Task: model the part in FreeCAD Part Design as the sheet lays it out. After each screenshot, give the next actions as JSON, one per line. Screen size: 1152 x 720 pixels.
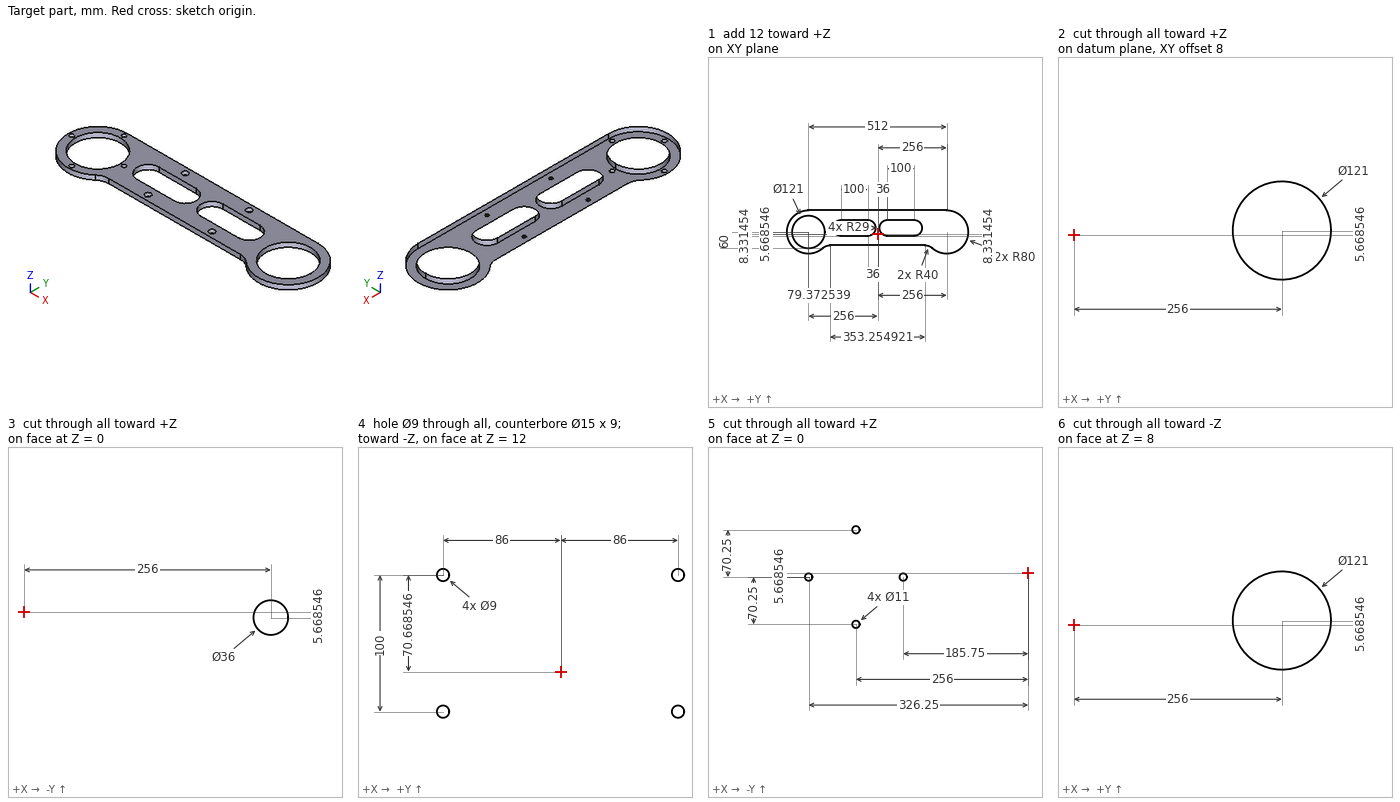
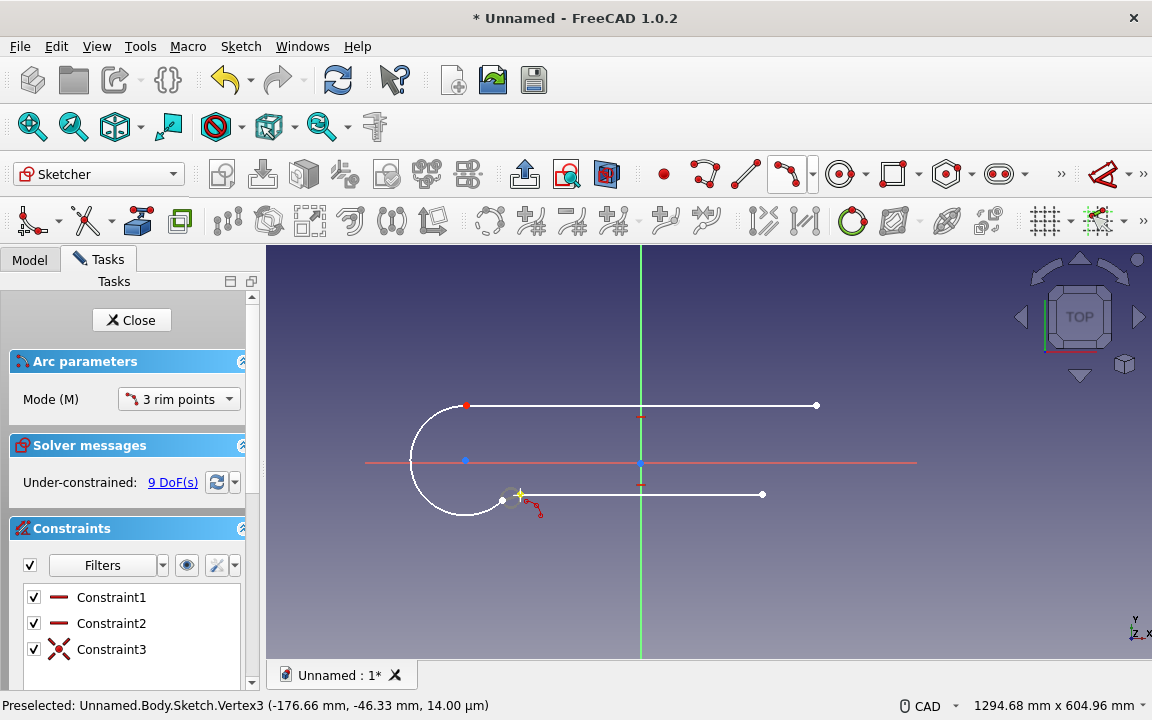
{"action": "scroll", "coordinate": [510, 495], "scroll_direction": "up", "scroll_amount": 11}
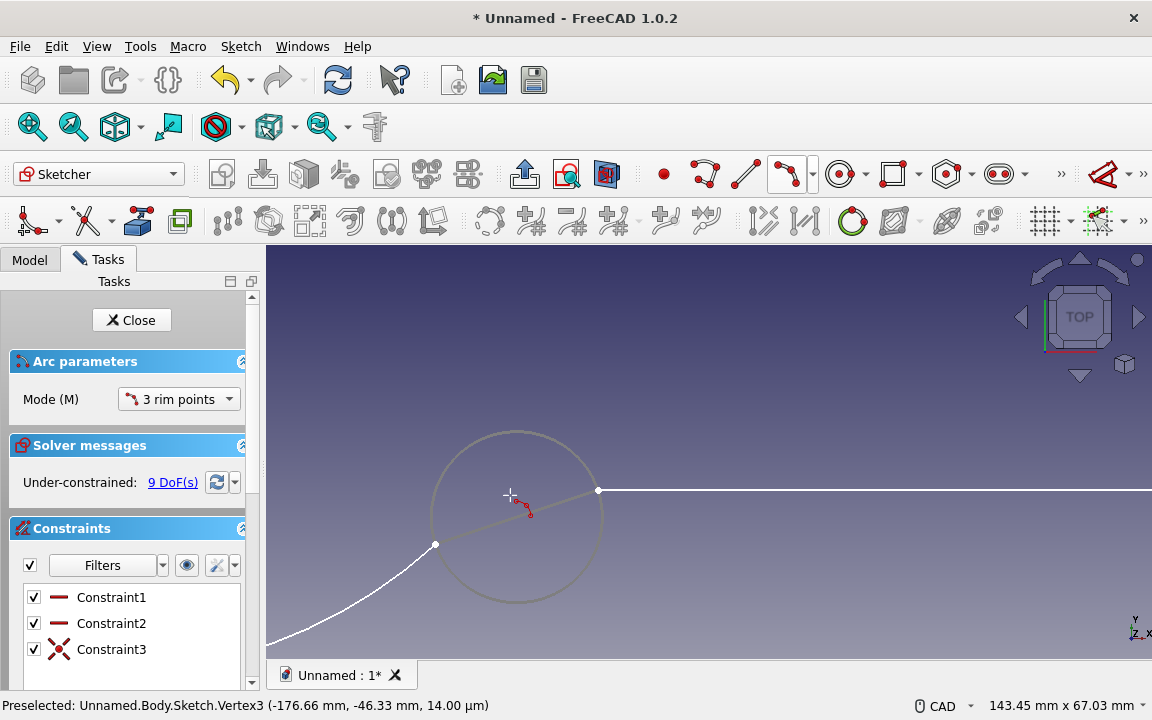
{"action": "left_click", "coordinate": [511, 494]}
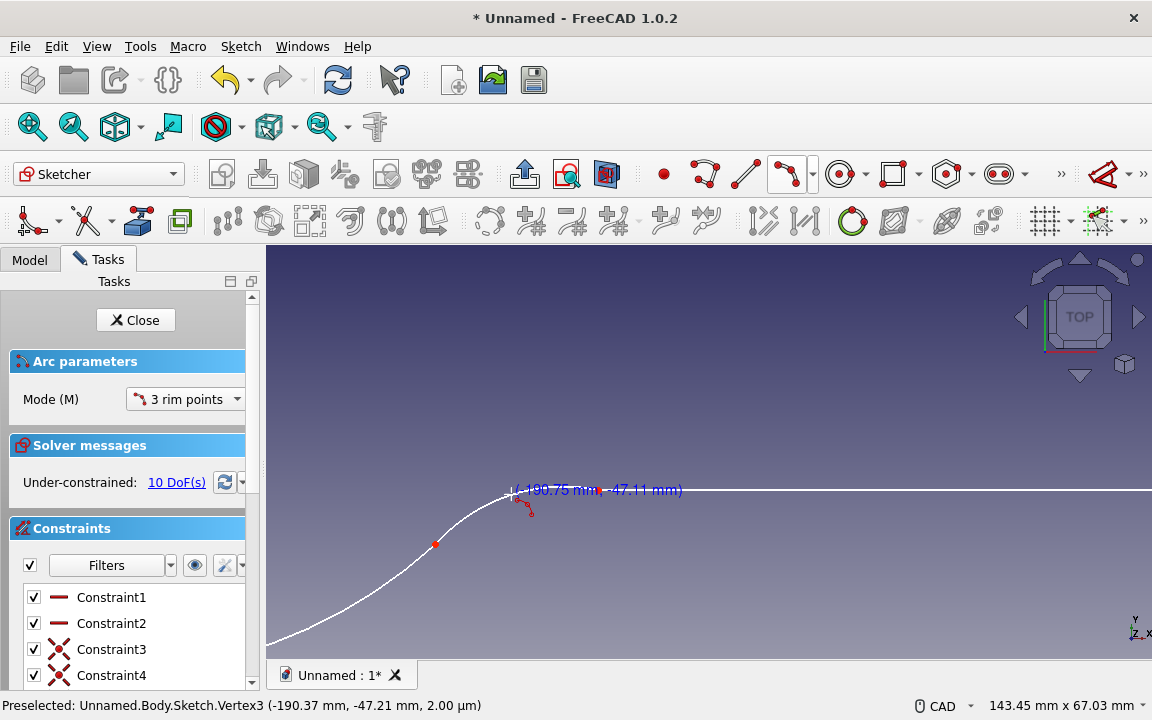
{"action": "scroll", "coordinate": [510, 495], "scroll_direction": "down", "scroll_amount": 11}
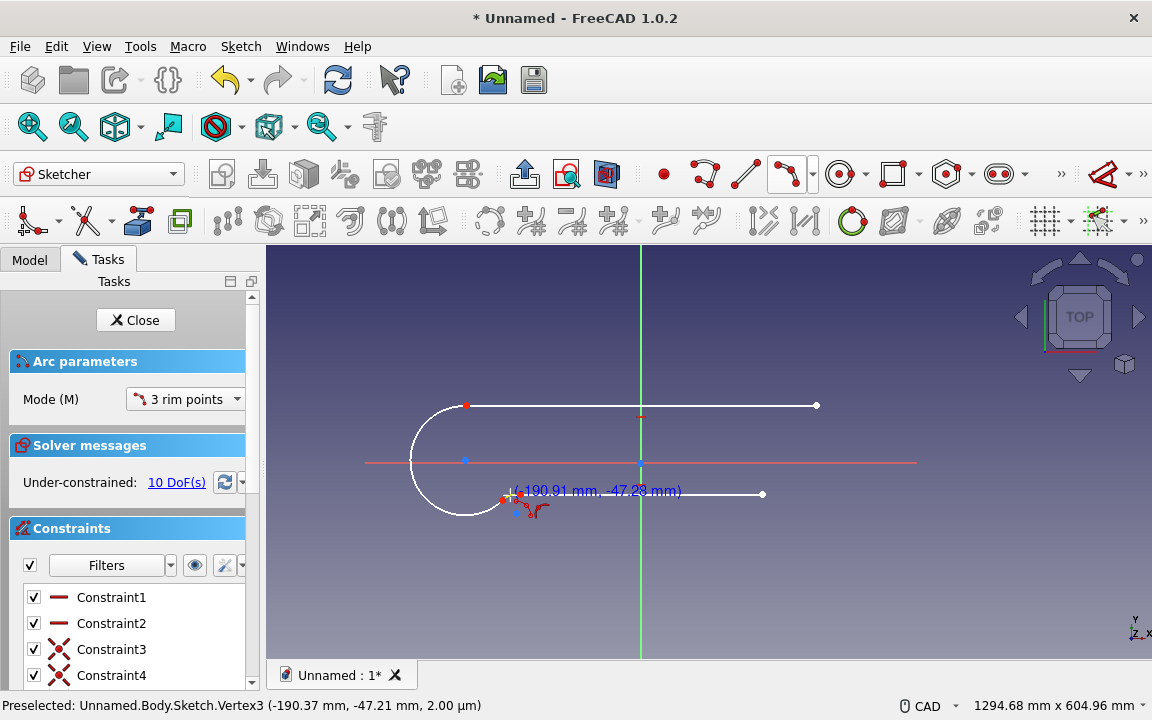
{"action": "left_click", "coordinate": [762, 495]}
{"action": "left_click", "coordinate": [780, 500]}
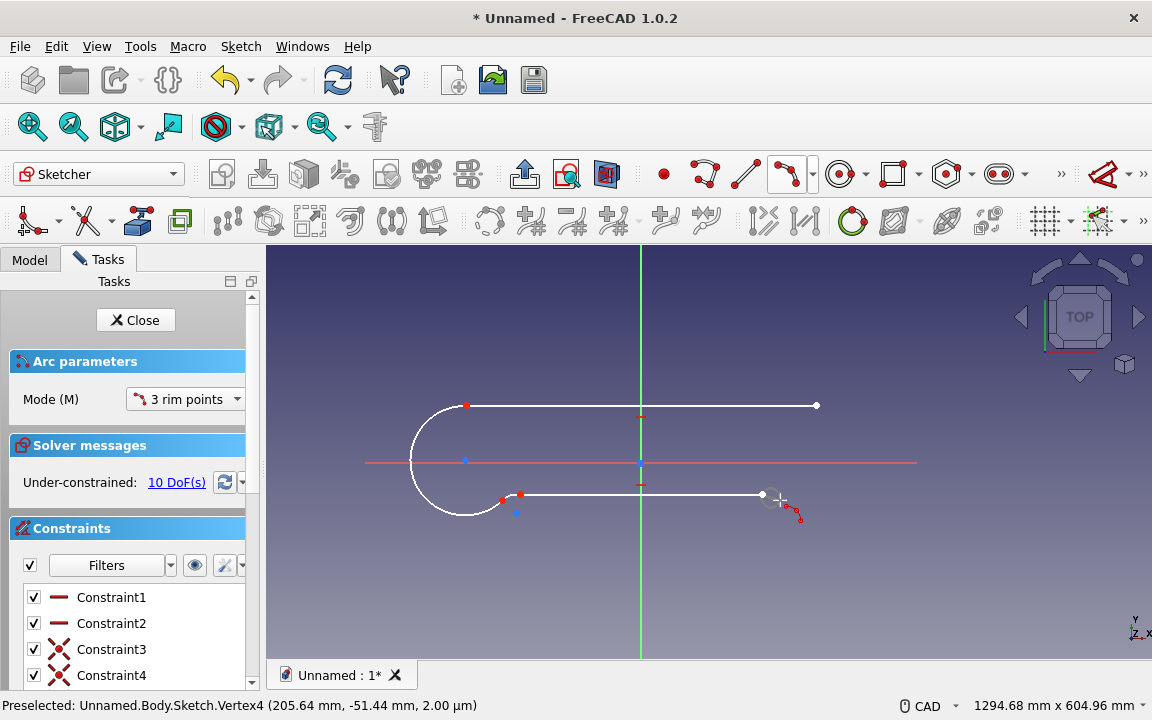
{"action": "scroll", "coordinate": [771, 495], "scroll_direction": "up", "scroll_amount": 11}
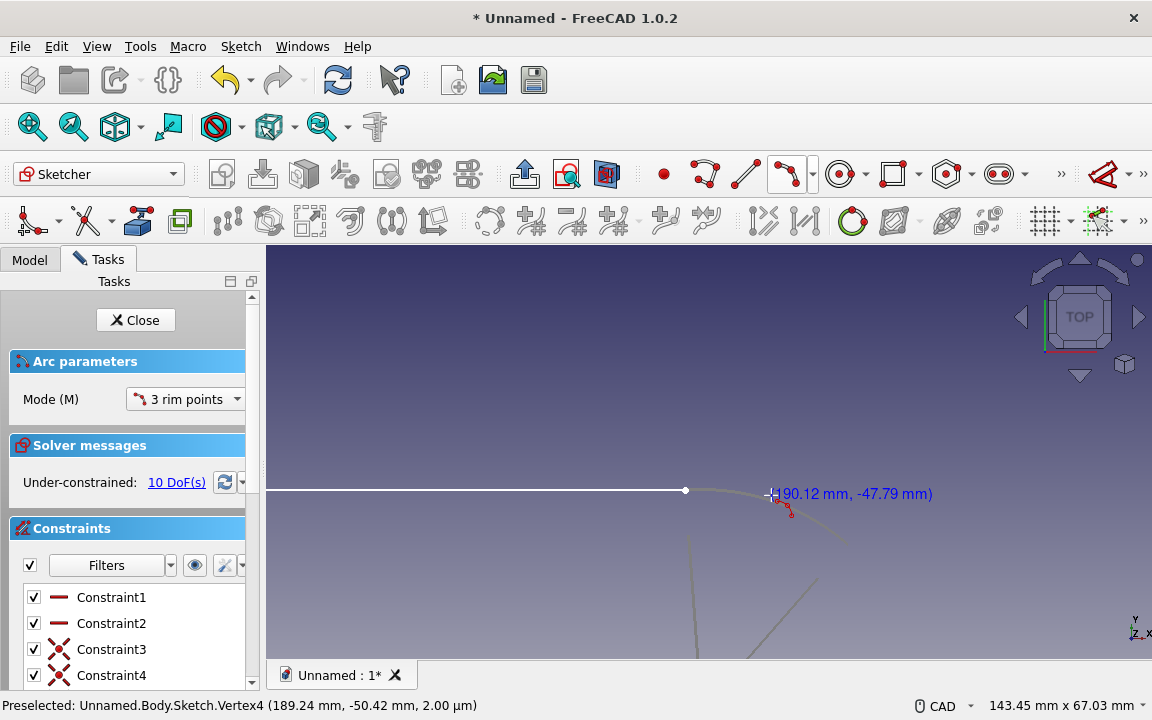
{"action": "left_click", "coordinate": [770, 494]}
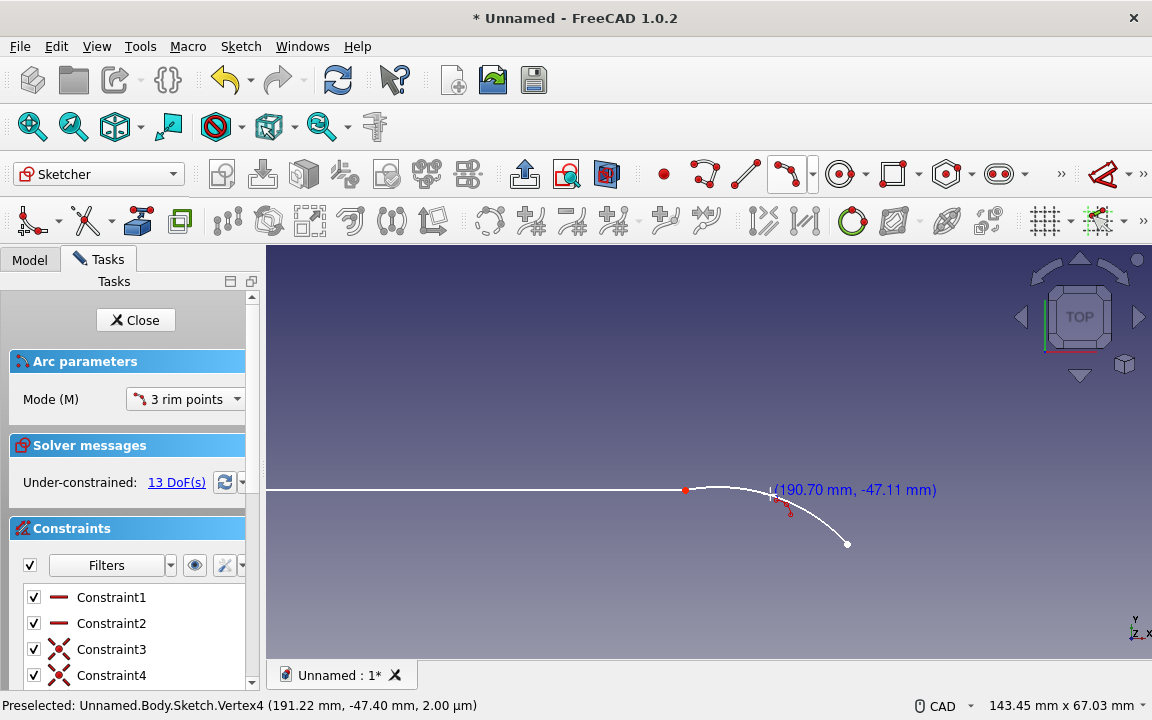
{"action": "scroll", "coordinate": [771, 495], "scroll_direction": "down", "scroll_amount": 11}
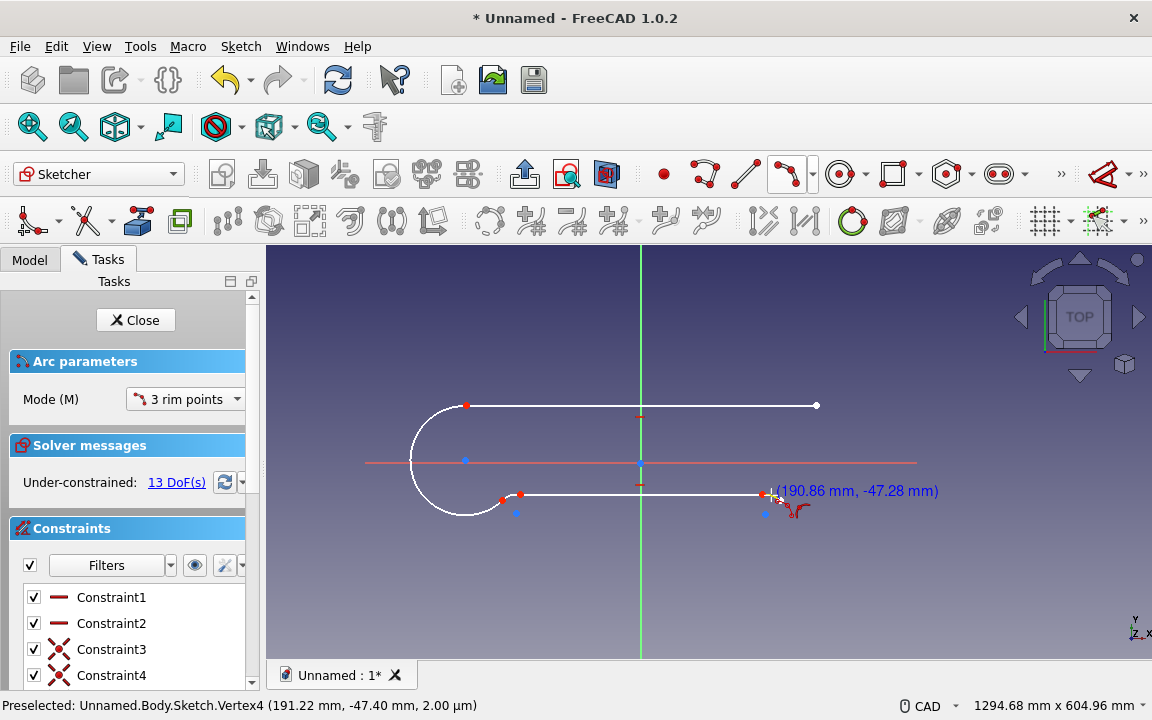
{"action": "left_click", "coordinate": [780, 501]}
{"action": "left_click", "coordinate": [816, 406]}
{"action": "left_click", "coordinate": [867, 479]}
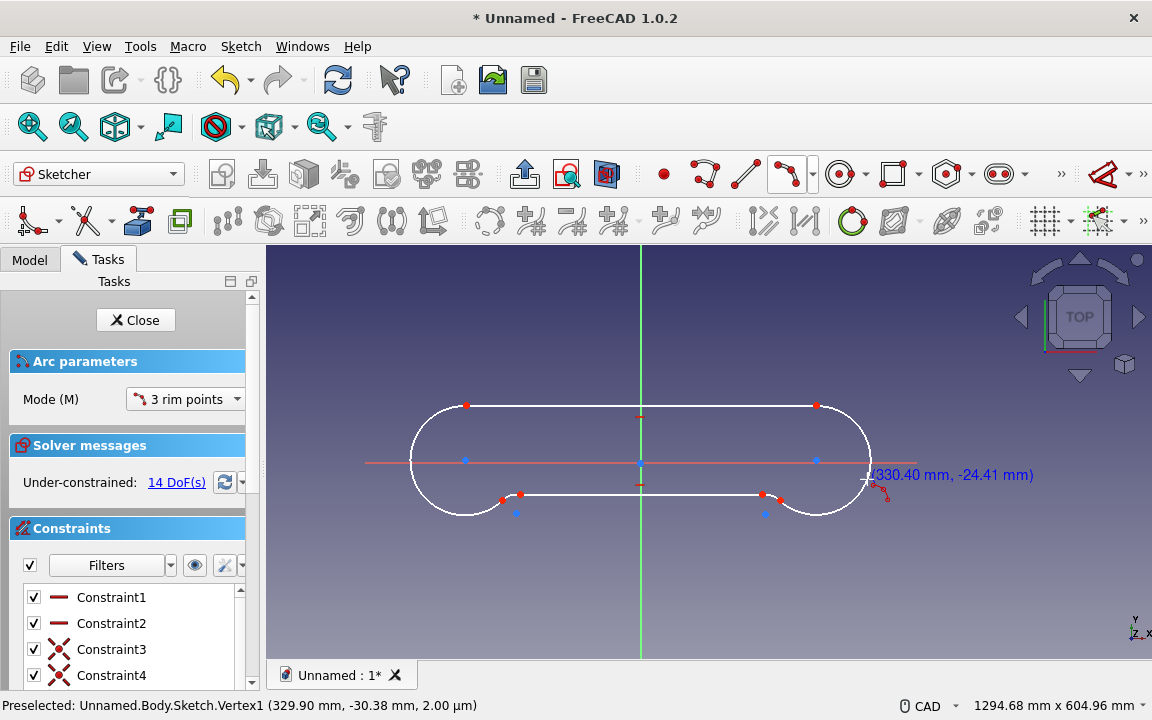
{"action": "left_click", "coordinate": [998, 174]}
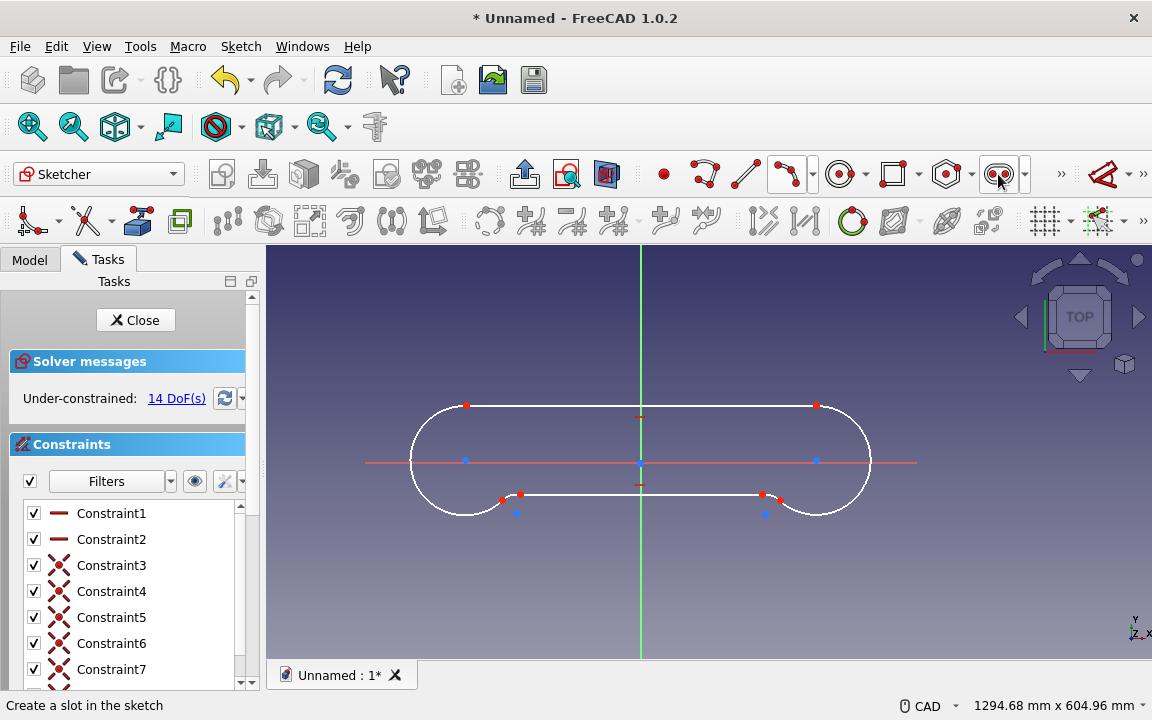
{"action": "left_click", "coordinate": [666, 449]}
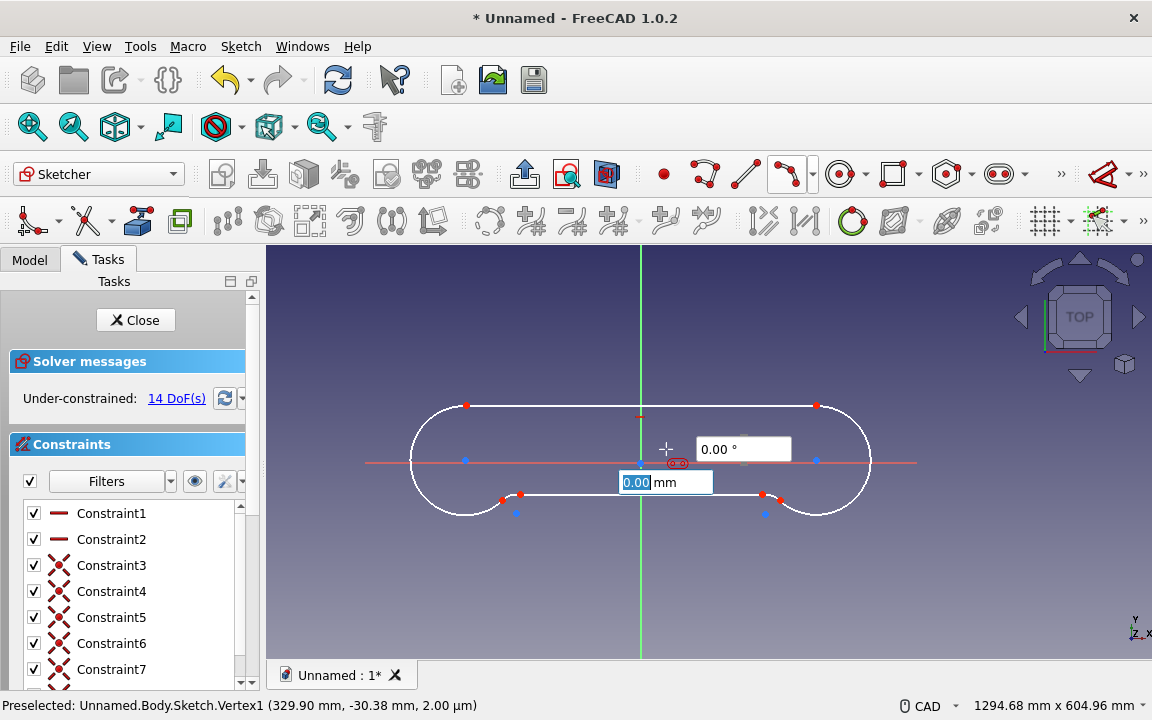
{"action": "left_click", "coordinate": [734, 449]}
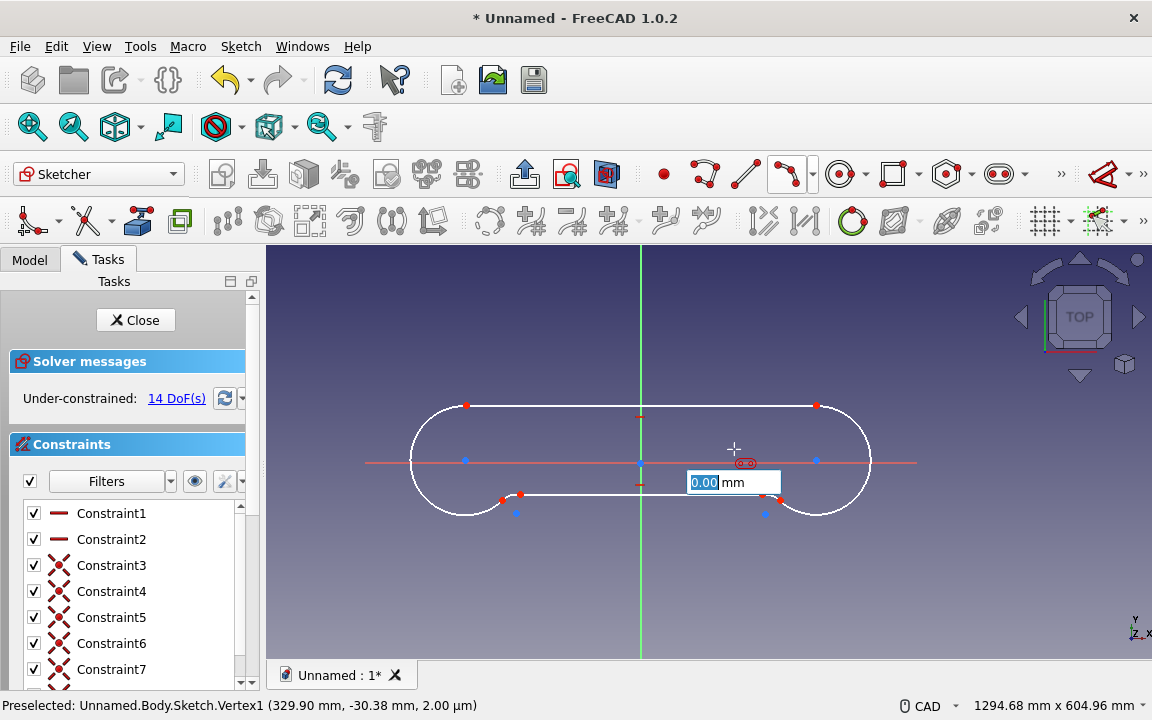
{"action": "left_click", "coordinate": [700, 429]}